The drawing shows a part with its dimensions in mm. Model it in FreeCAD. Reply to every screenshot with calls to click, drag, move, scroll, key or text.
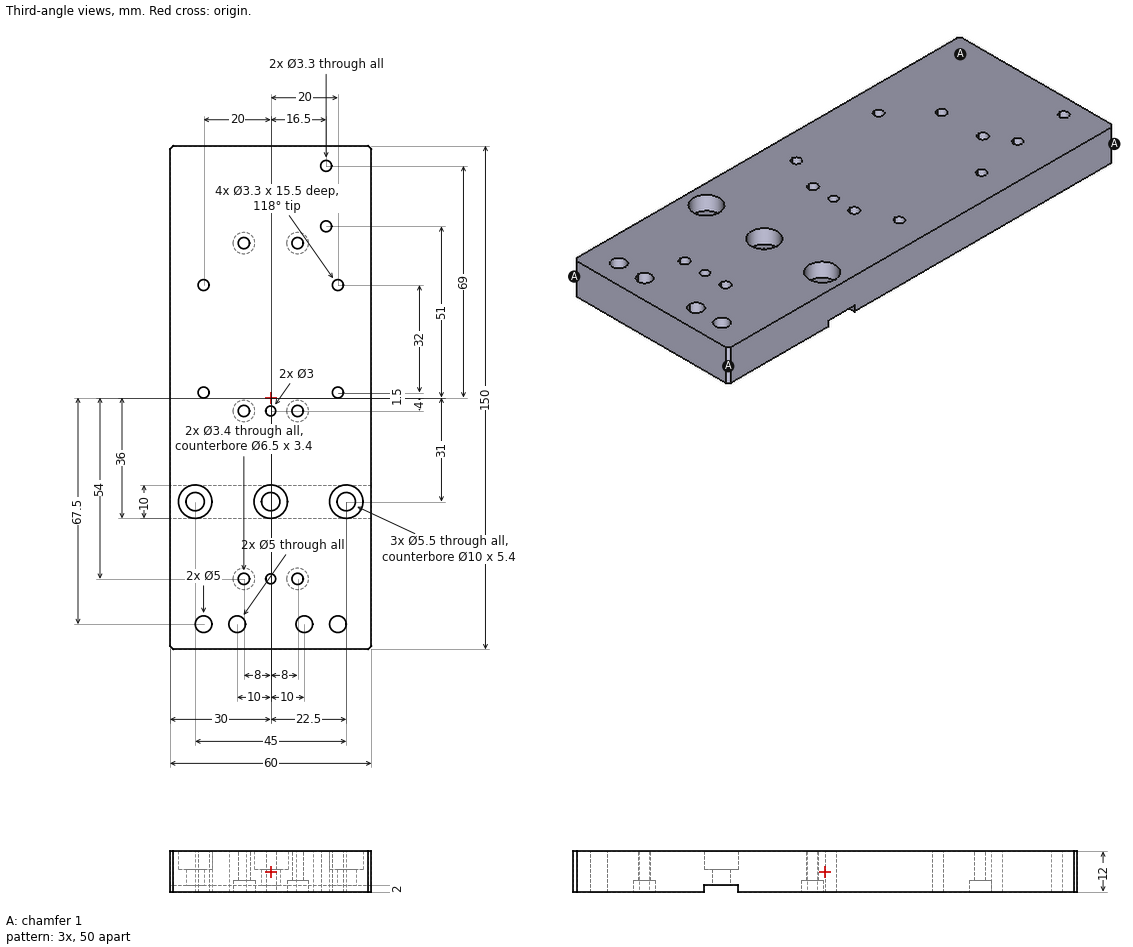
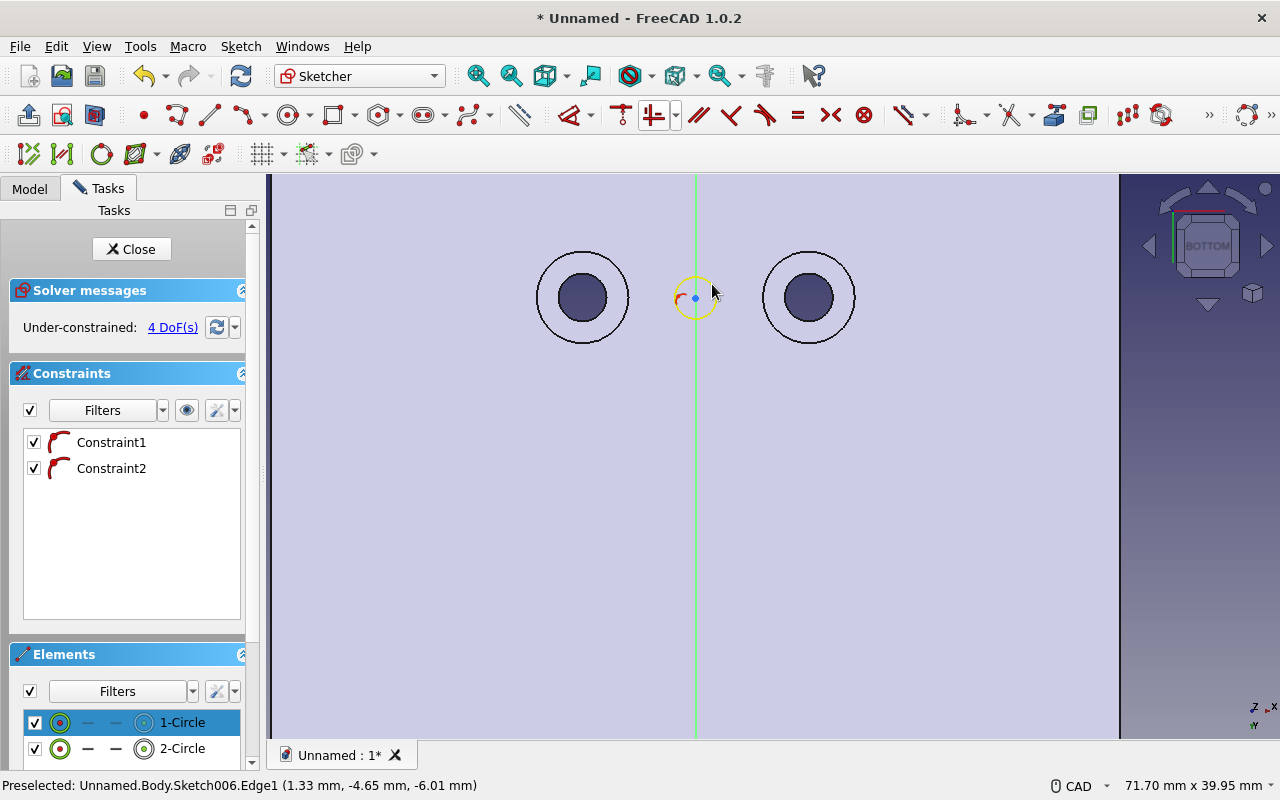
click(710, 283)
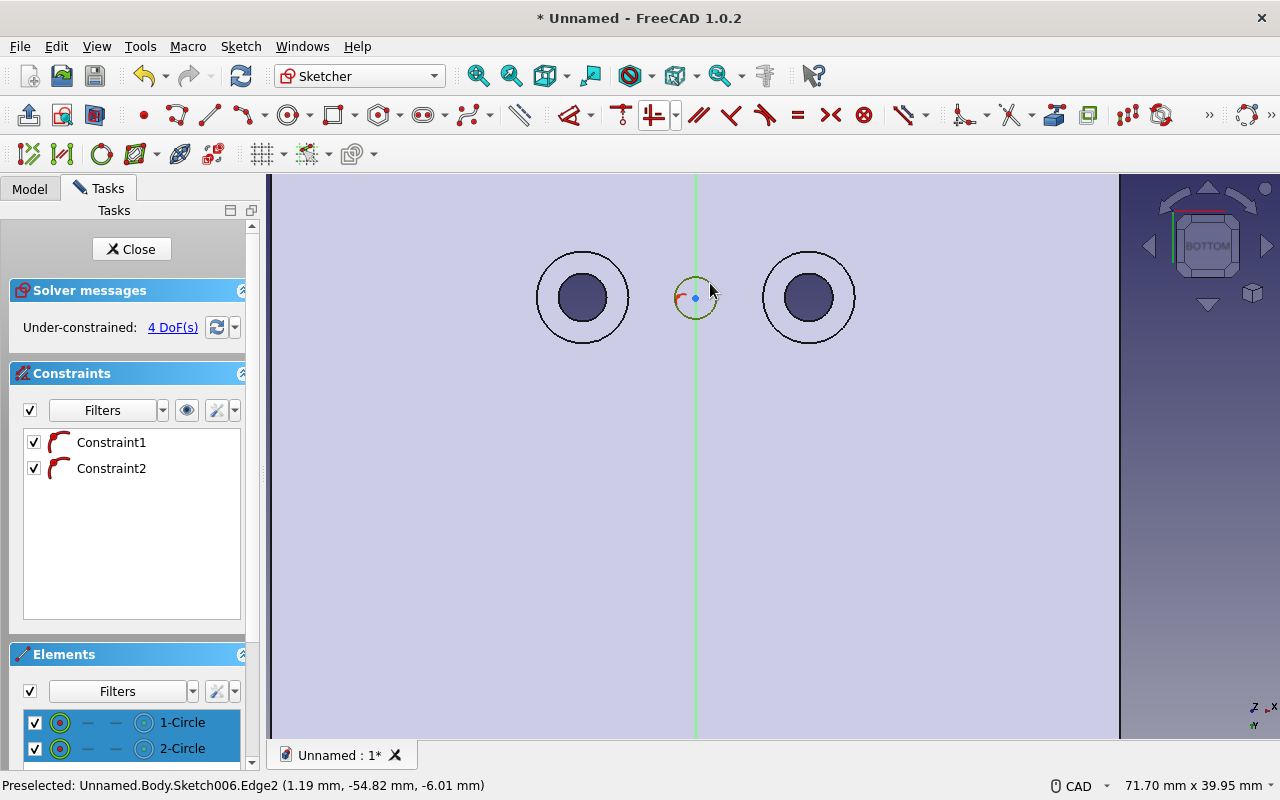
click(798, 116)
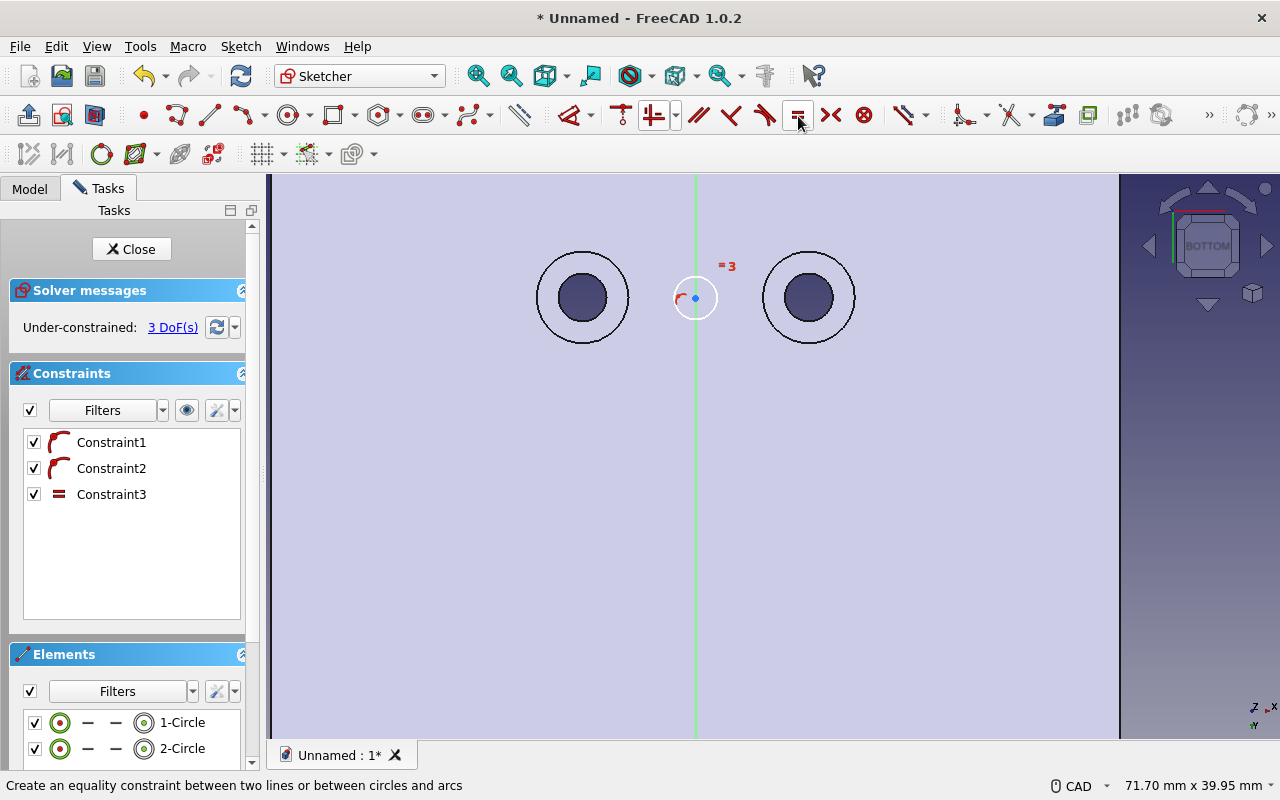
click(568, 116)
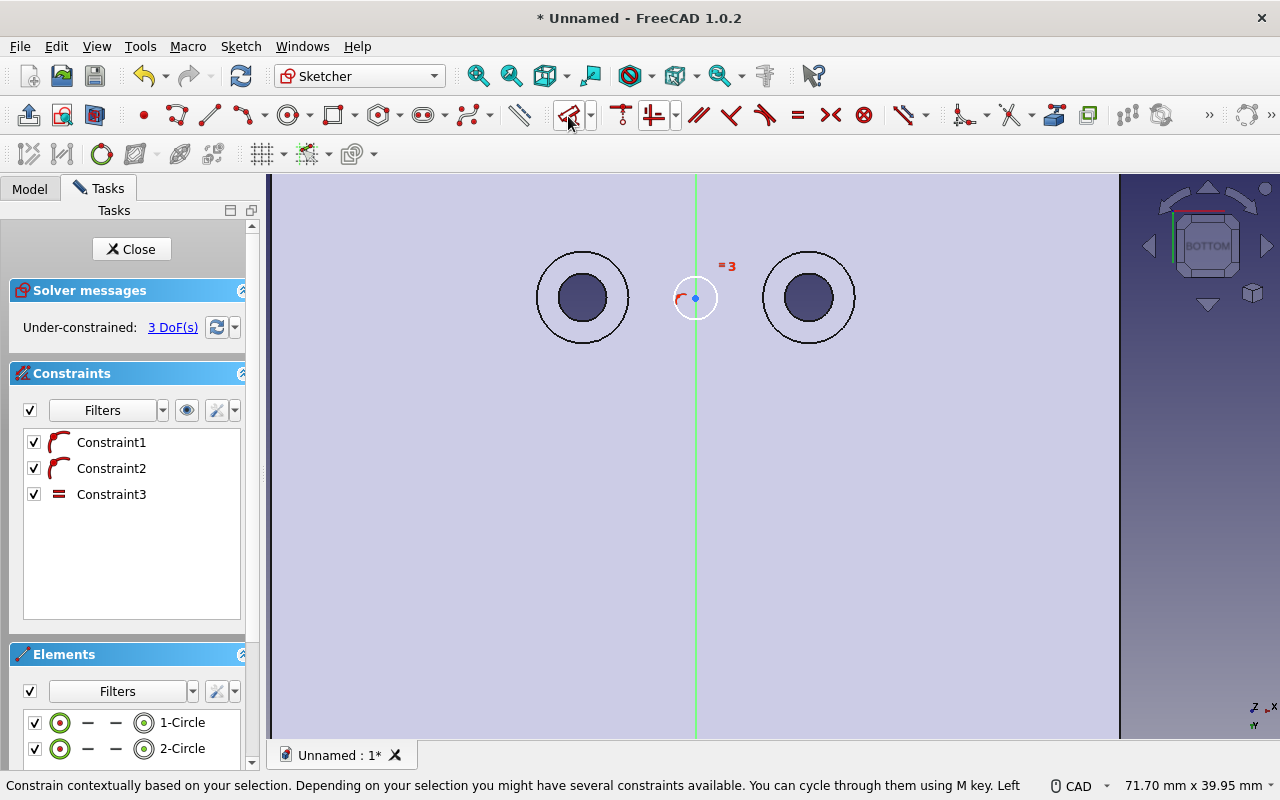
scroll(712, 283, down, 4)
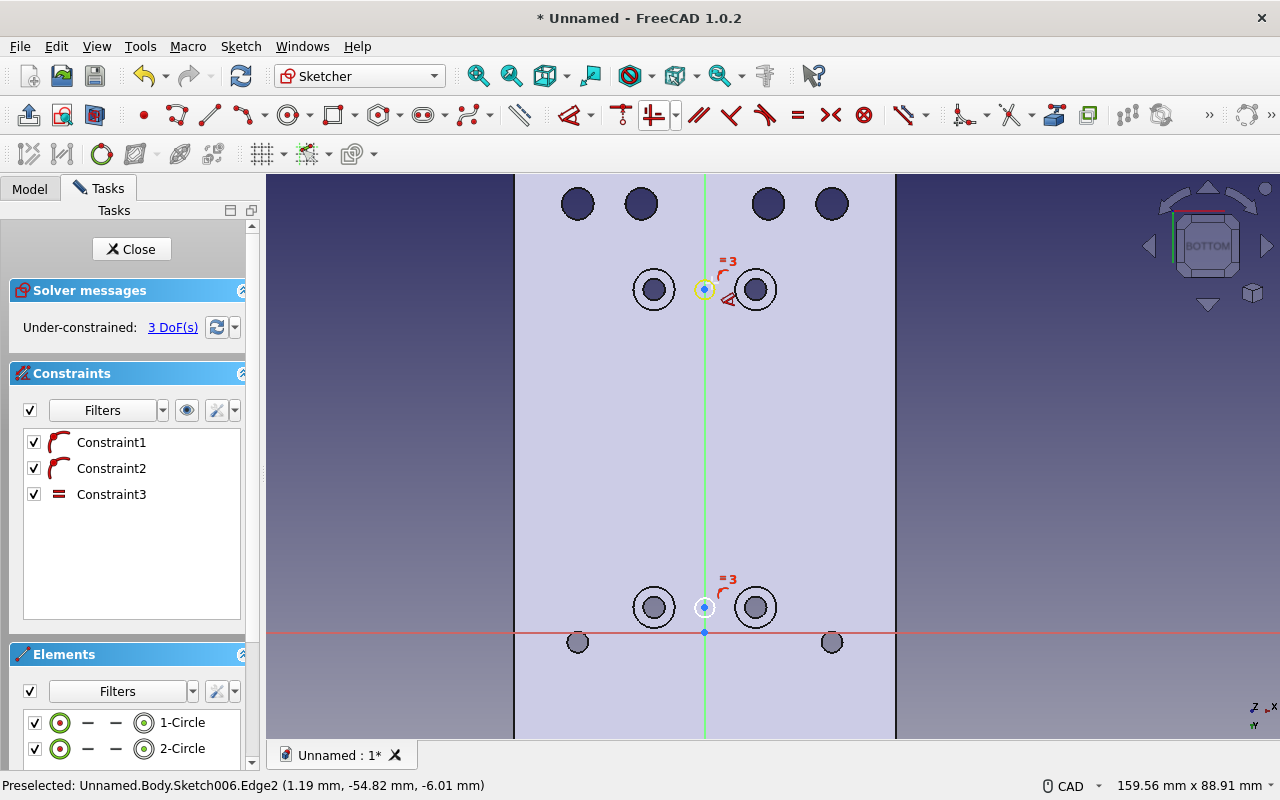
scroll(712, 601, up, 4)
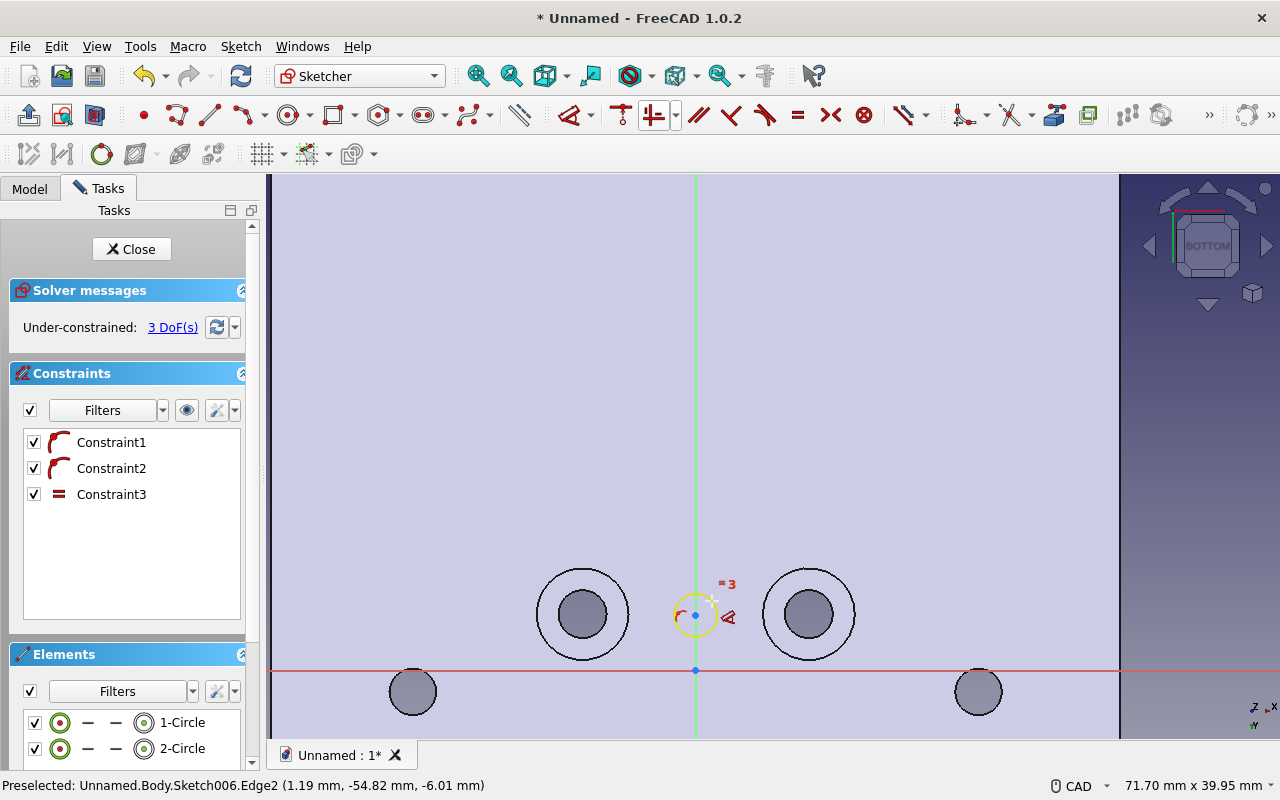
click(711, 600)
click(734, 577)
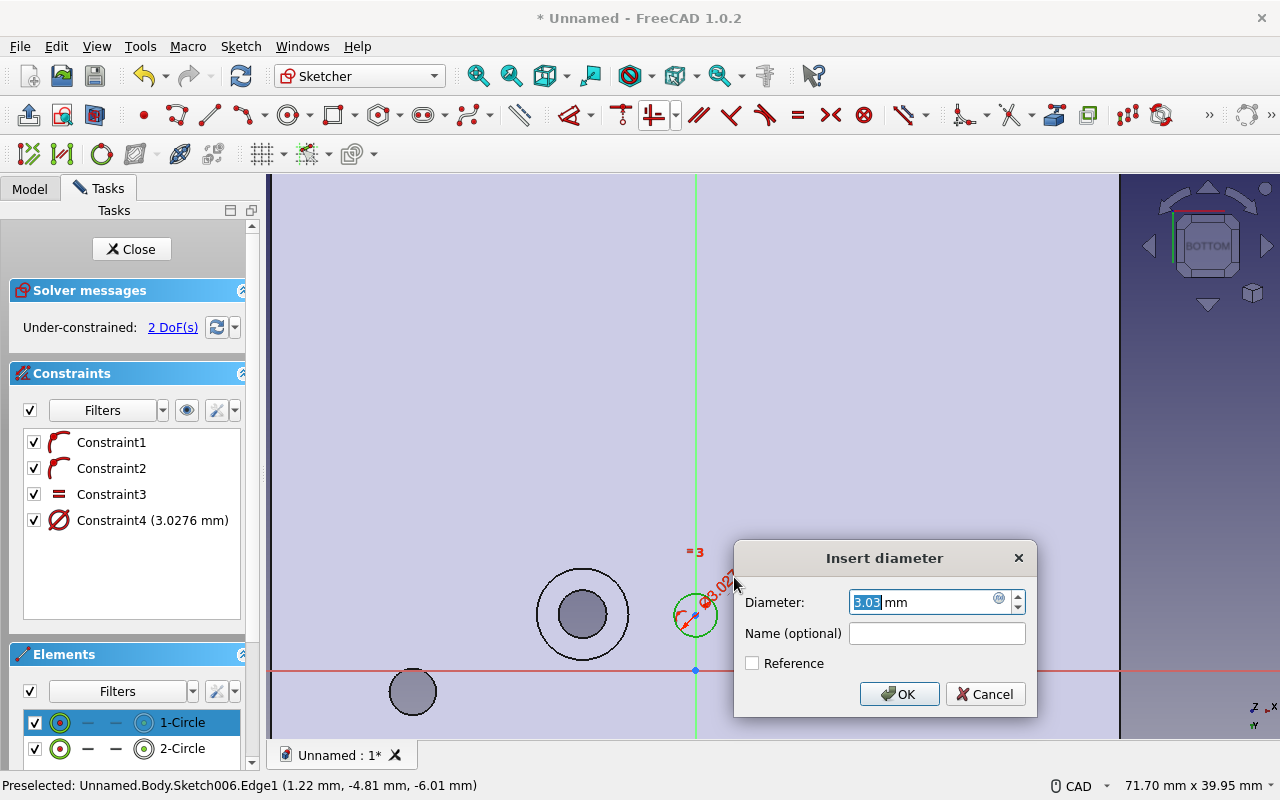
text(3)
key(Return)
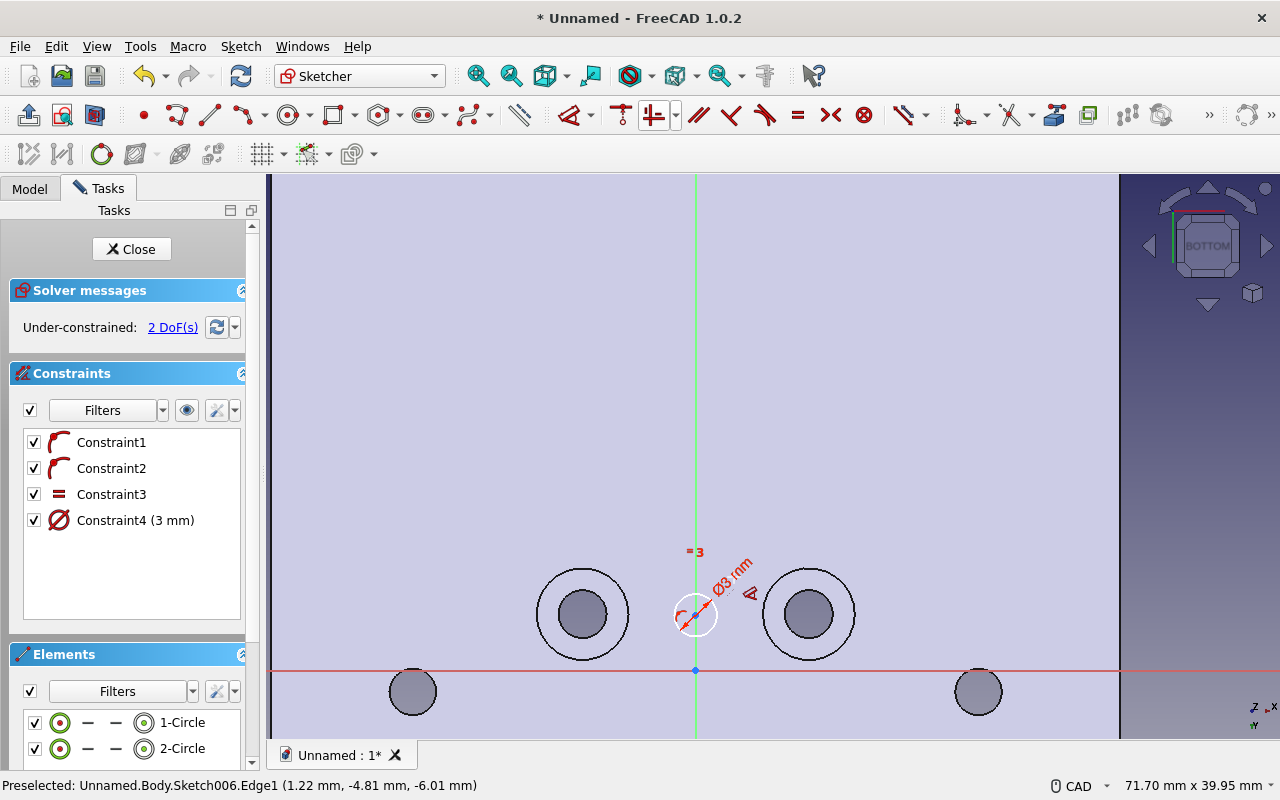
click(696, 615)
click(730, 643)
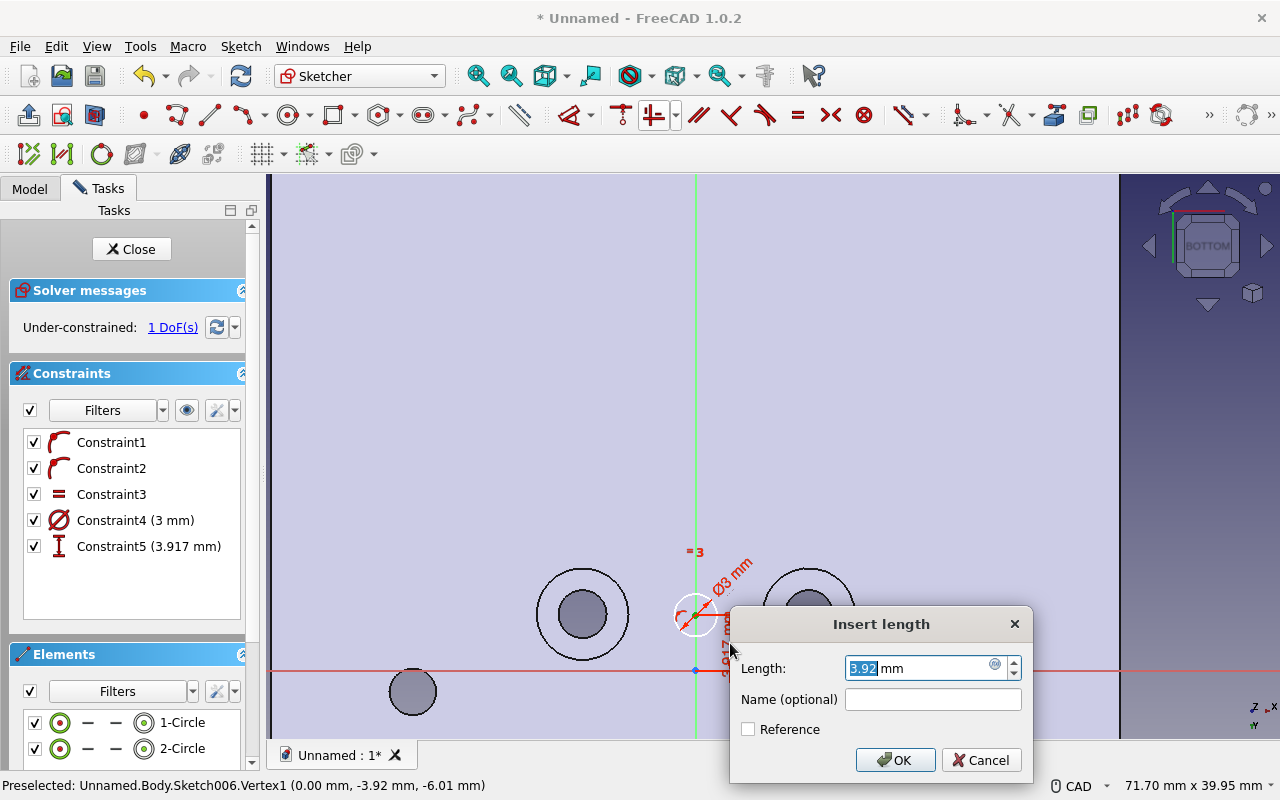
text(4)
key(Return)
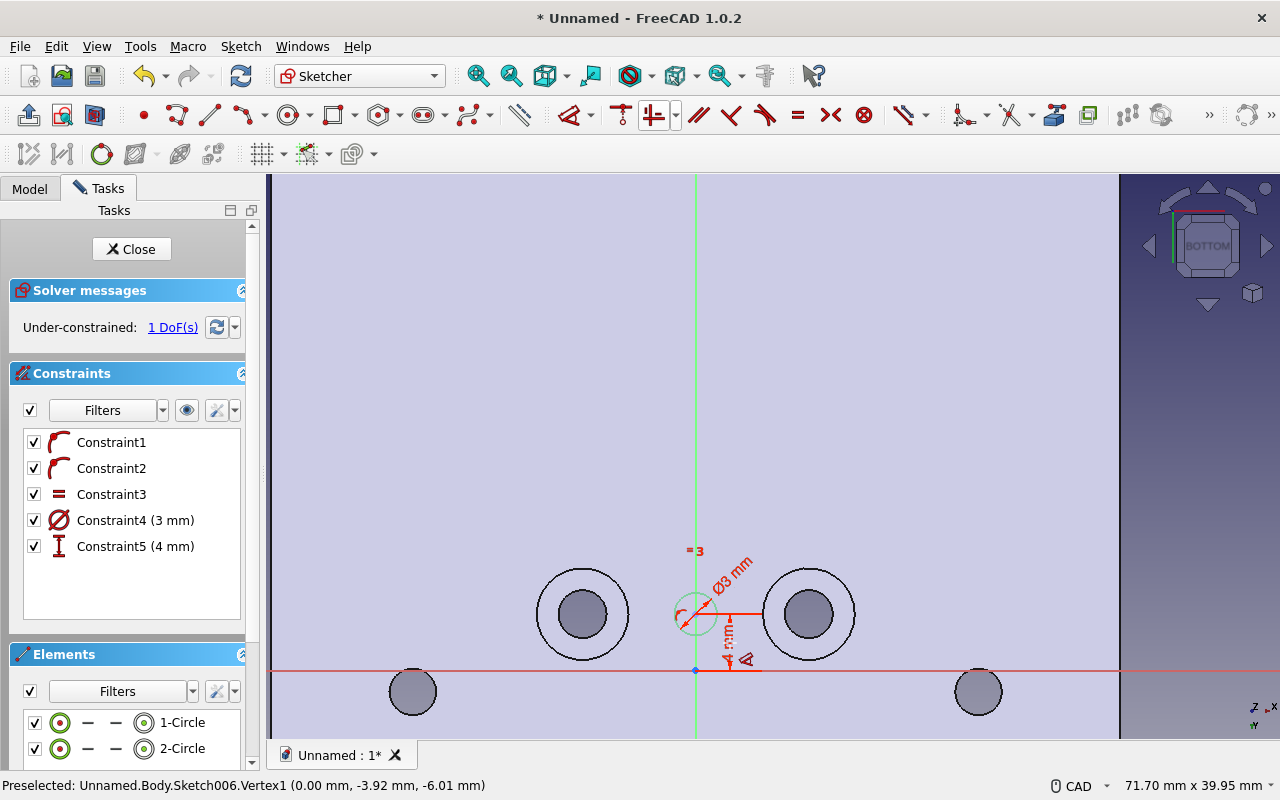
scroll(712, 602, down, 4)